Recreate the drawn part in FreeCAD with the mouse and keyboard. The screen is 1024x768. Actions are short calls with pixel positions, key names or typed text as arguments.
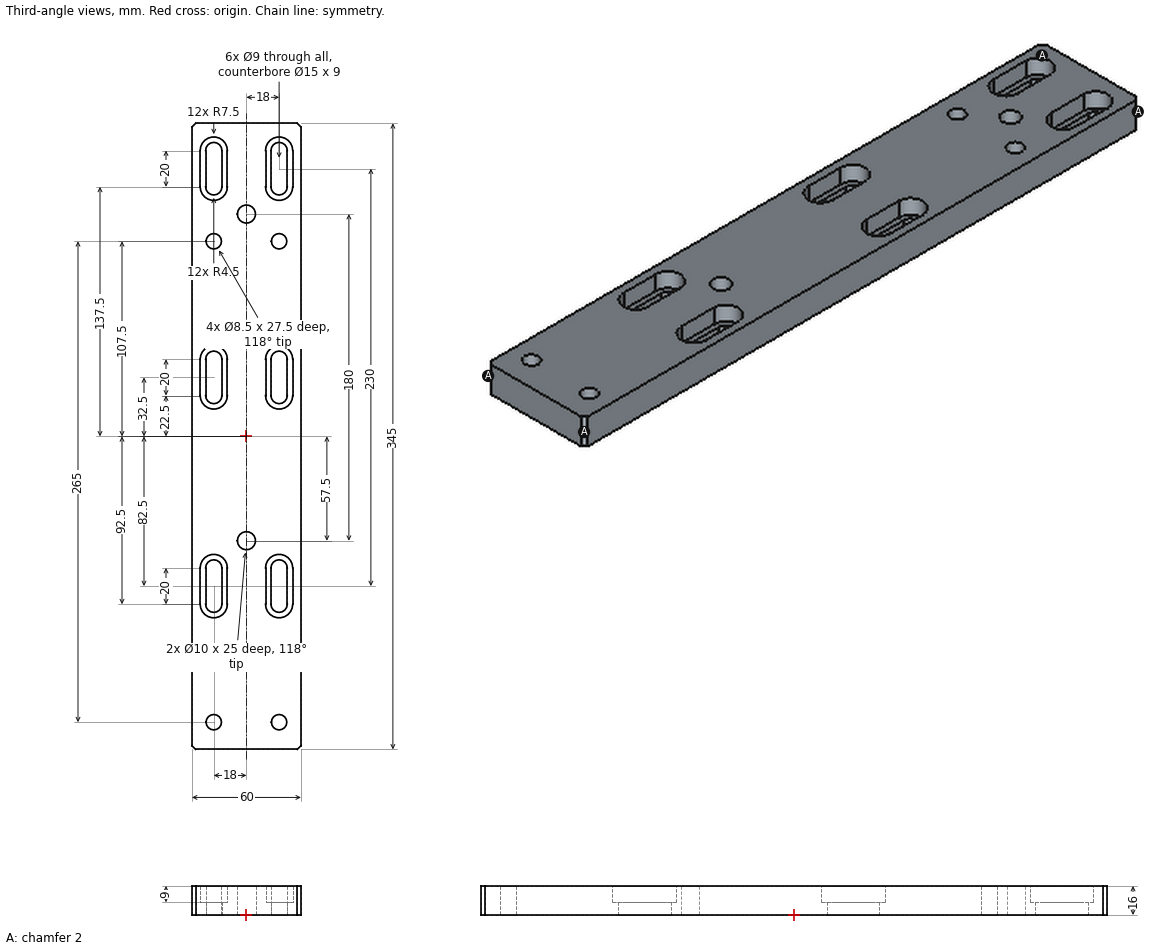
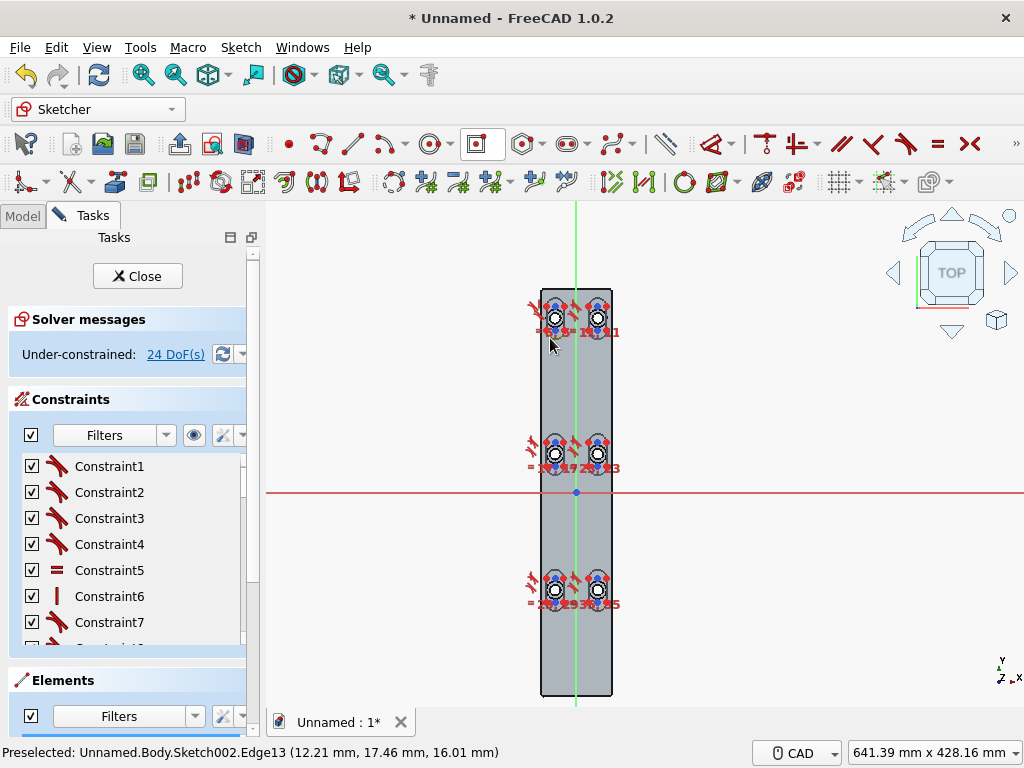
scroll(550, 609, up, 3)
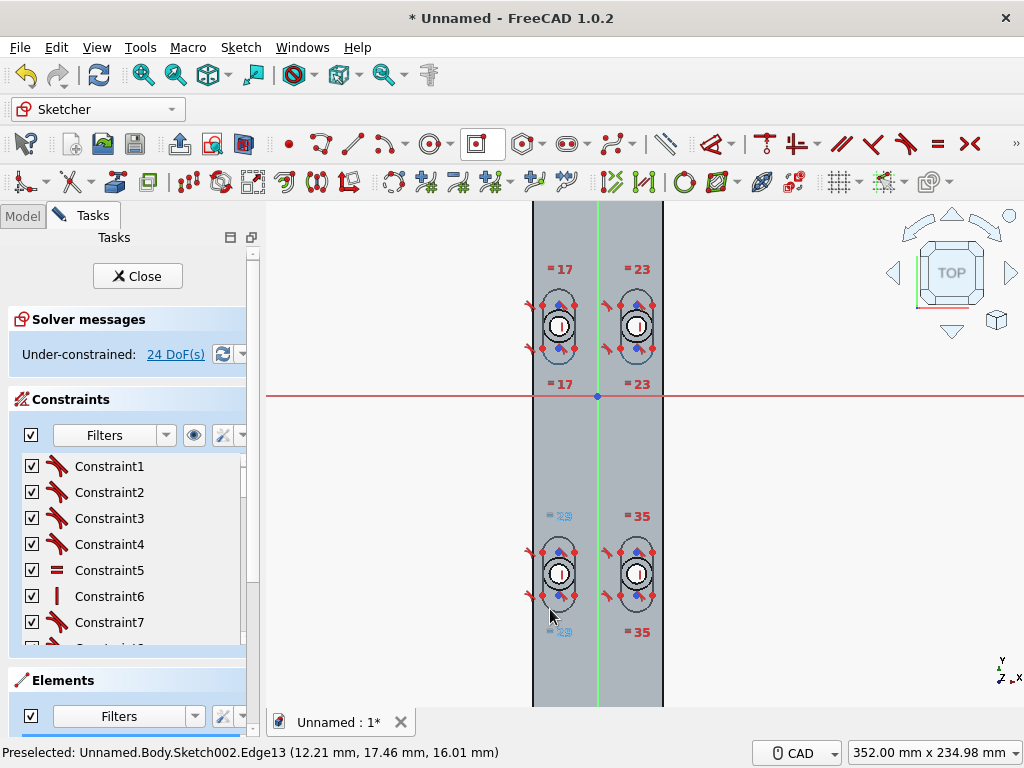
click(549, 609)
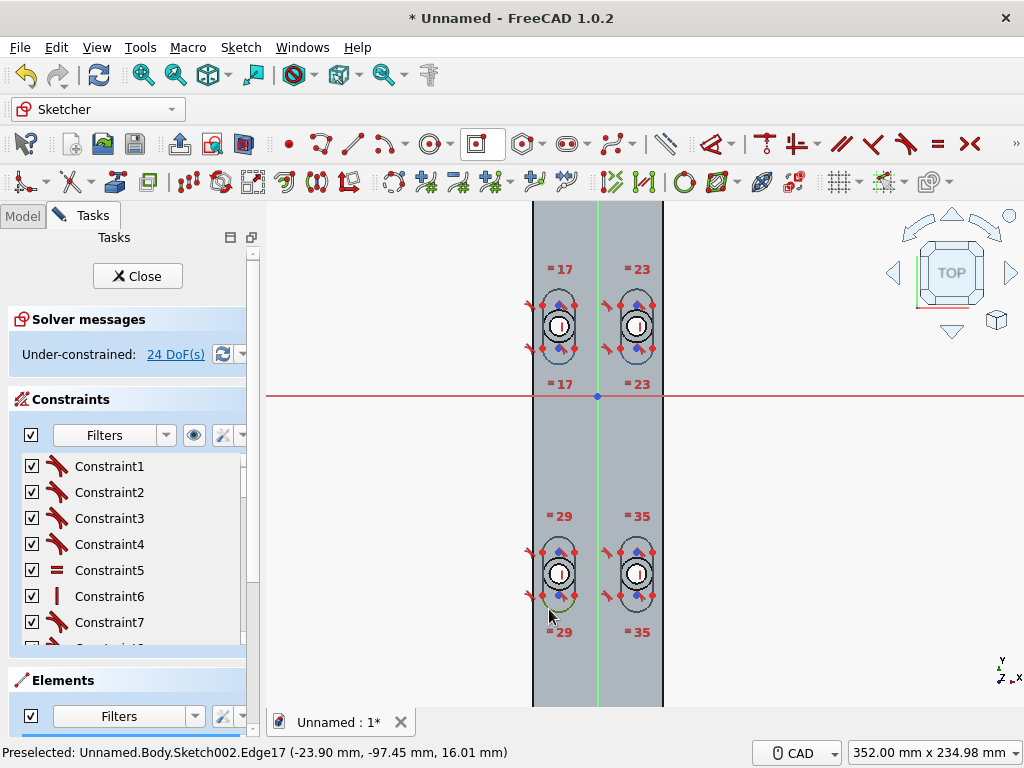
click(627, 609)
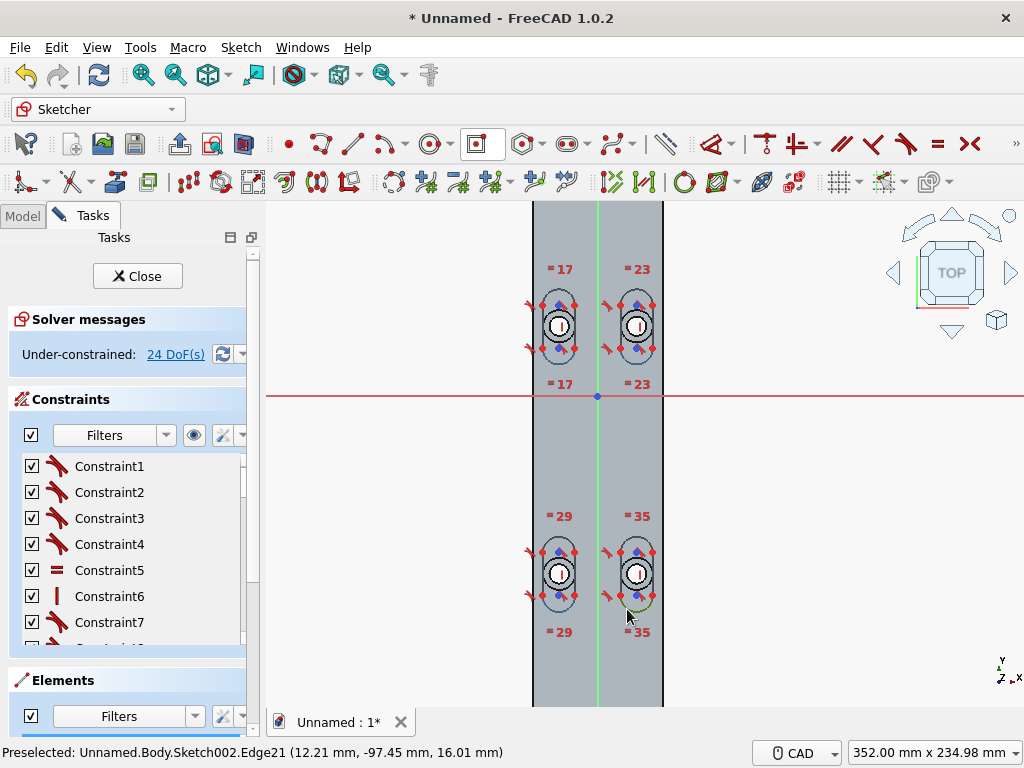
click(938, 144)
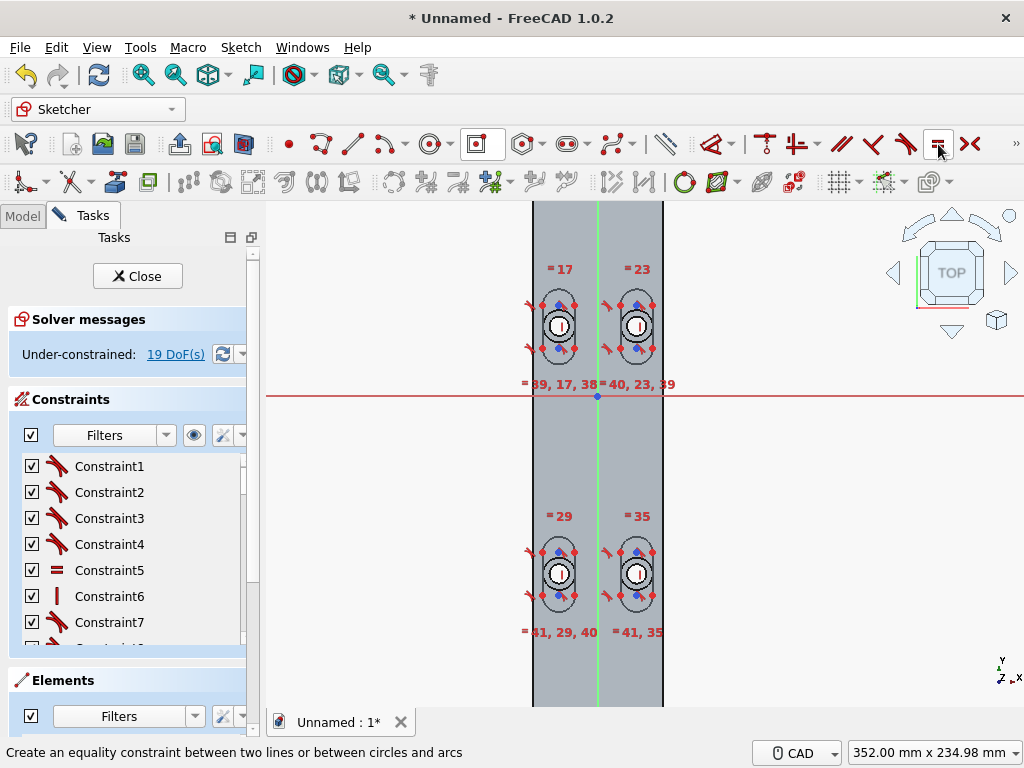
scroll(550, 609, down, 3)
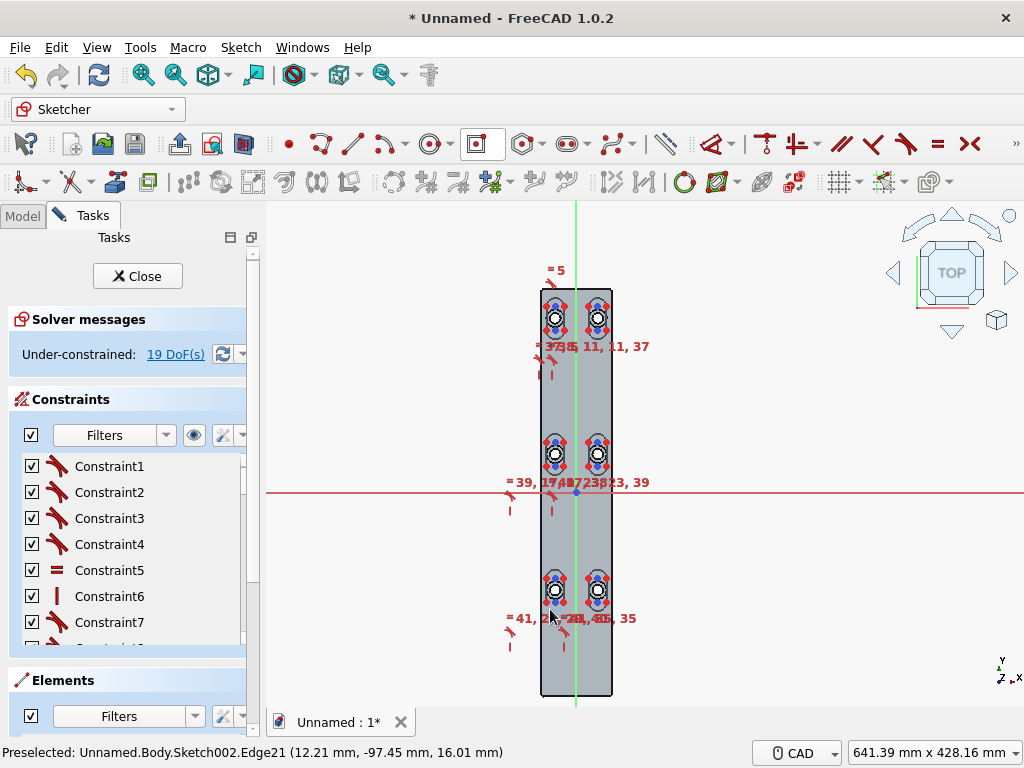
scroll(555, 331, up, 2)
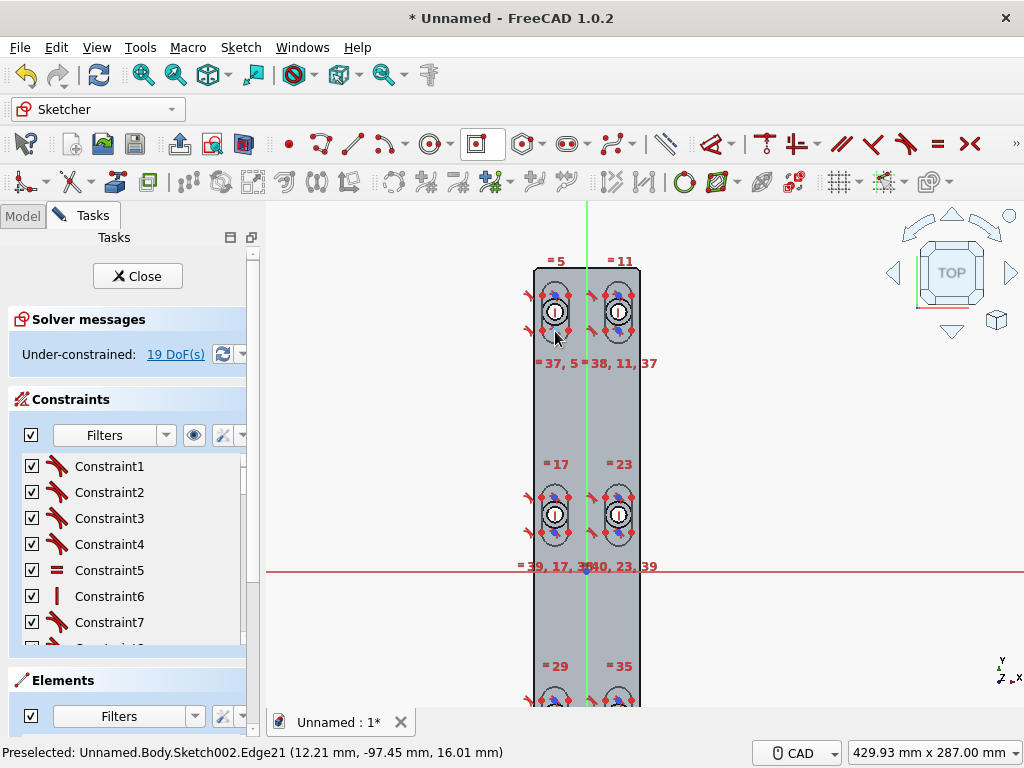
click(555, 330)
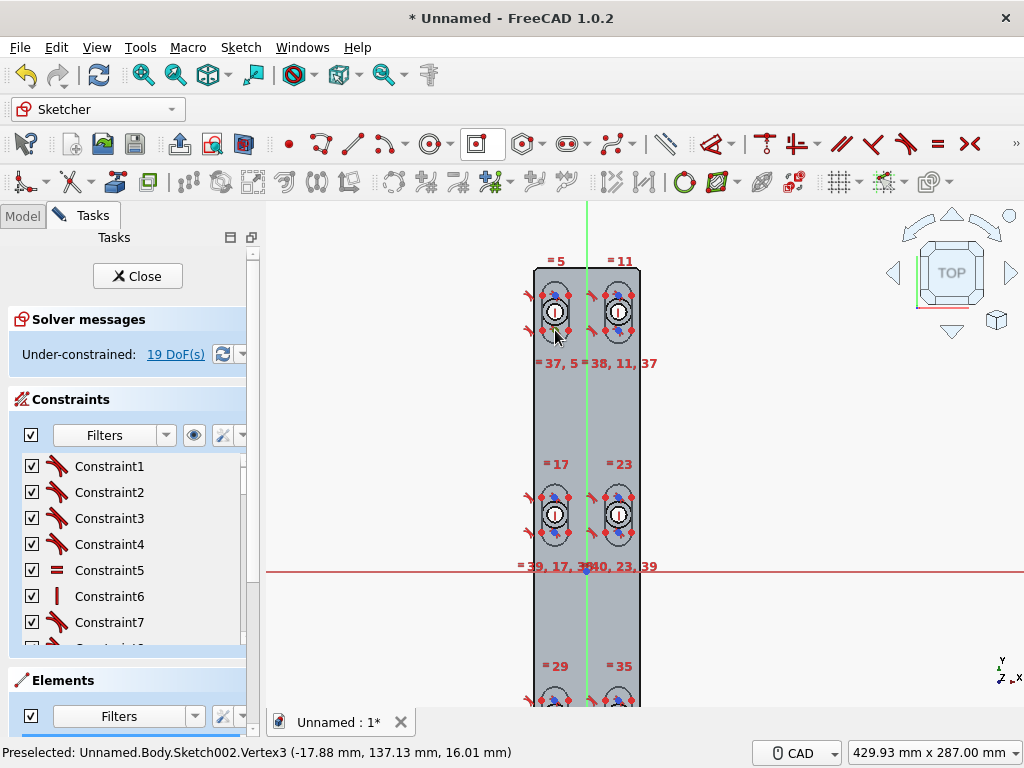
click(618, 330)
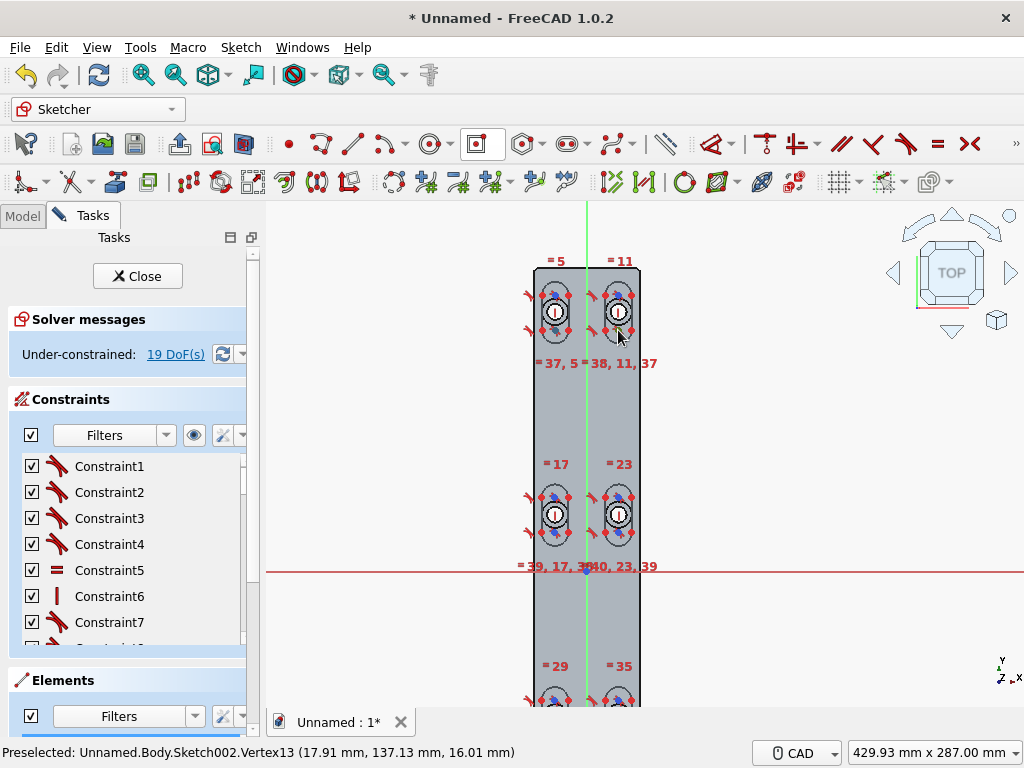
click(587, 647)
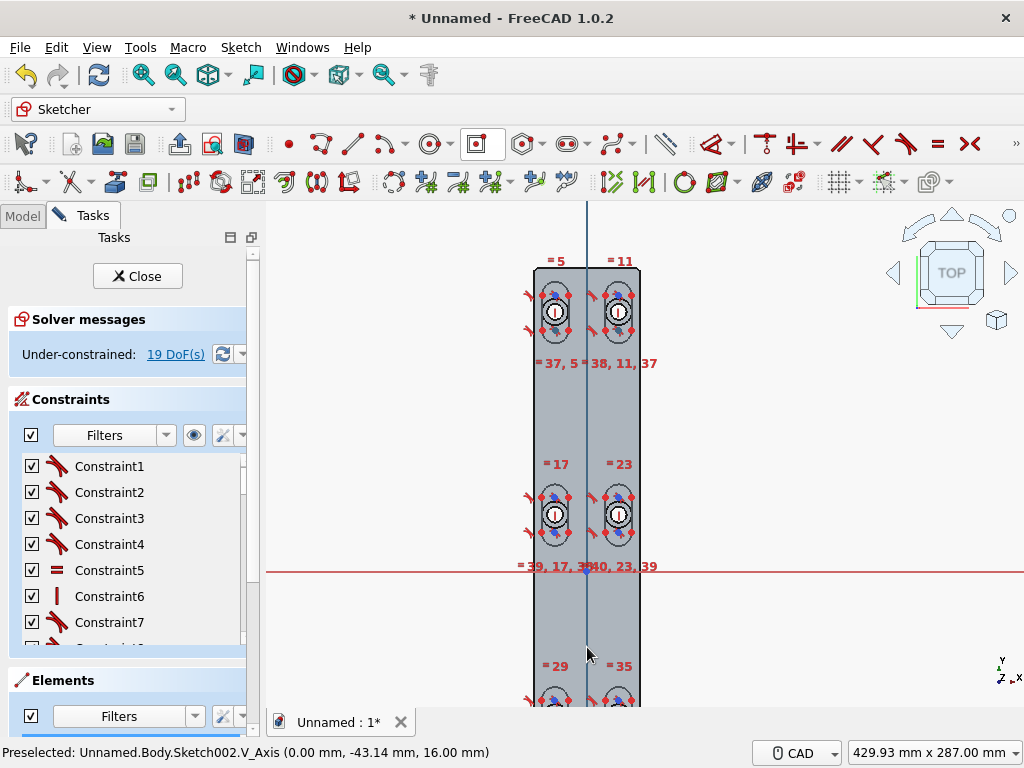
click(970, 144)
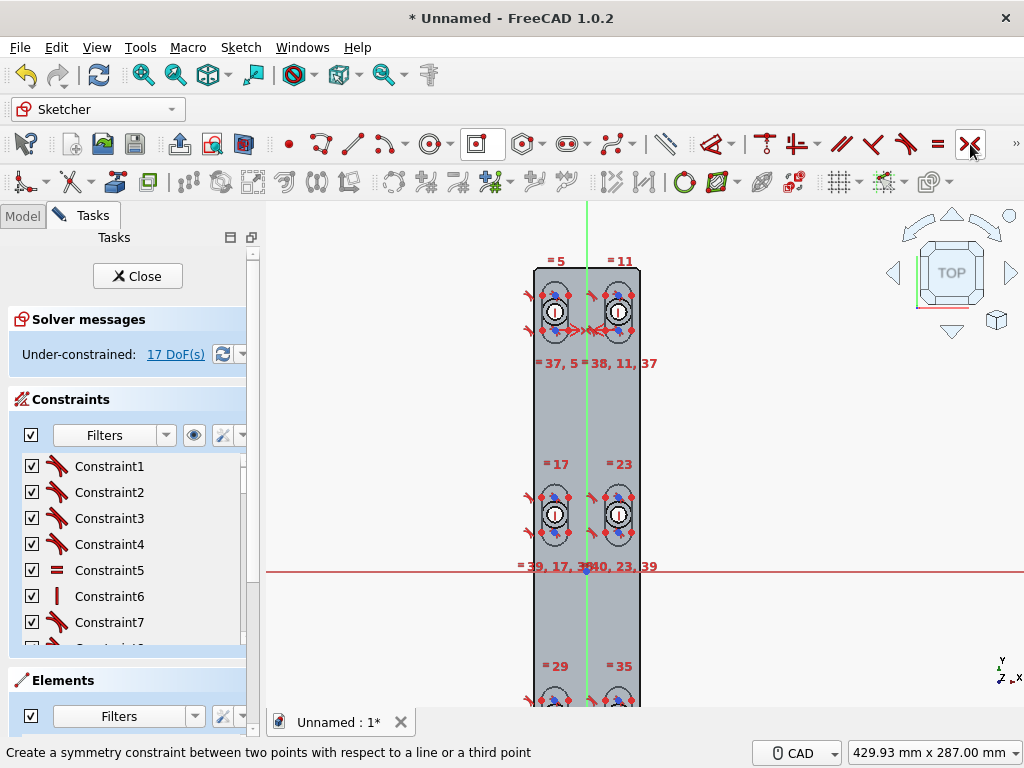
click(555, 533)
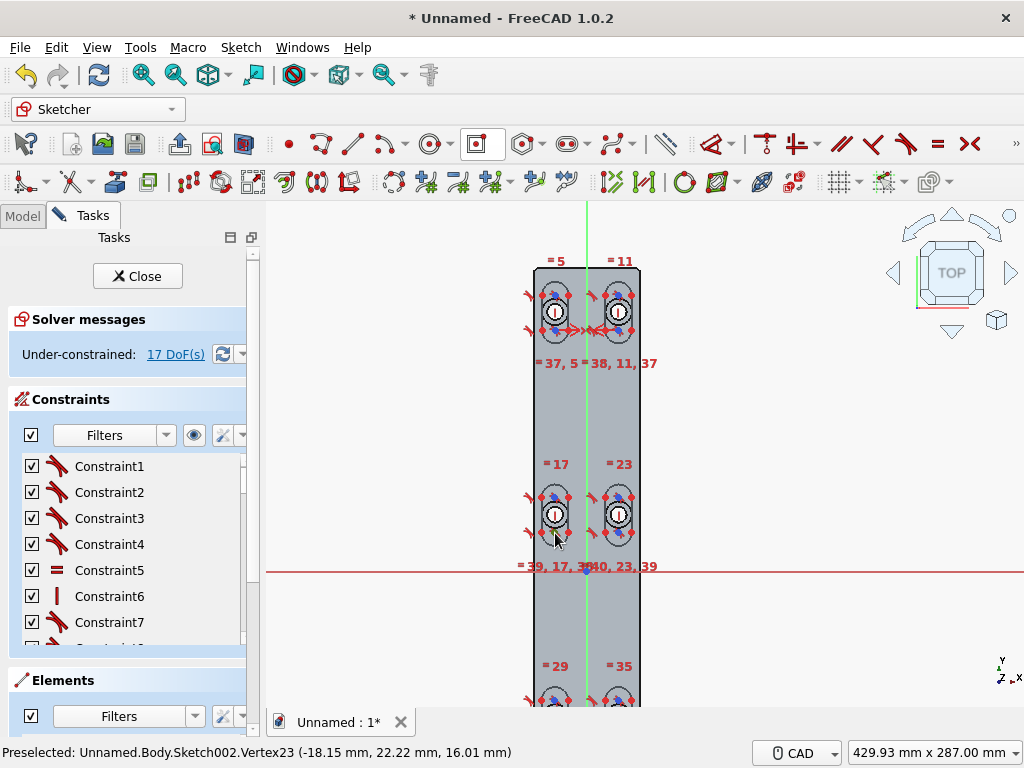
click(619, 533)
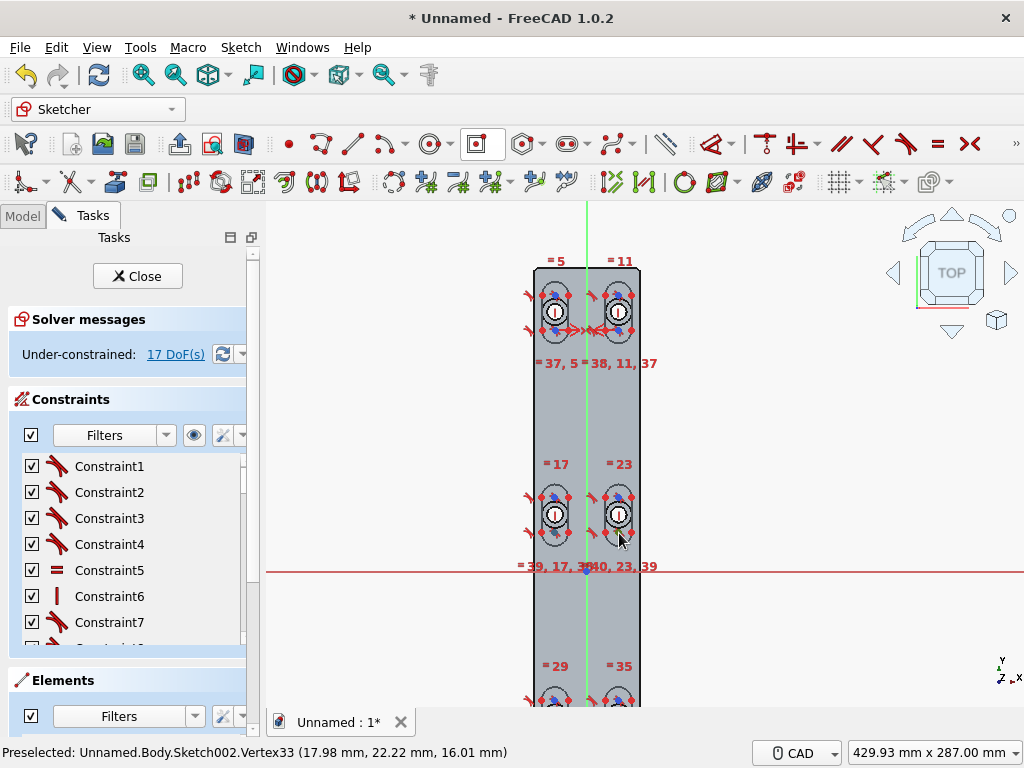
click(587, 647)